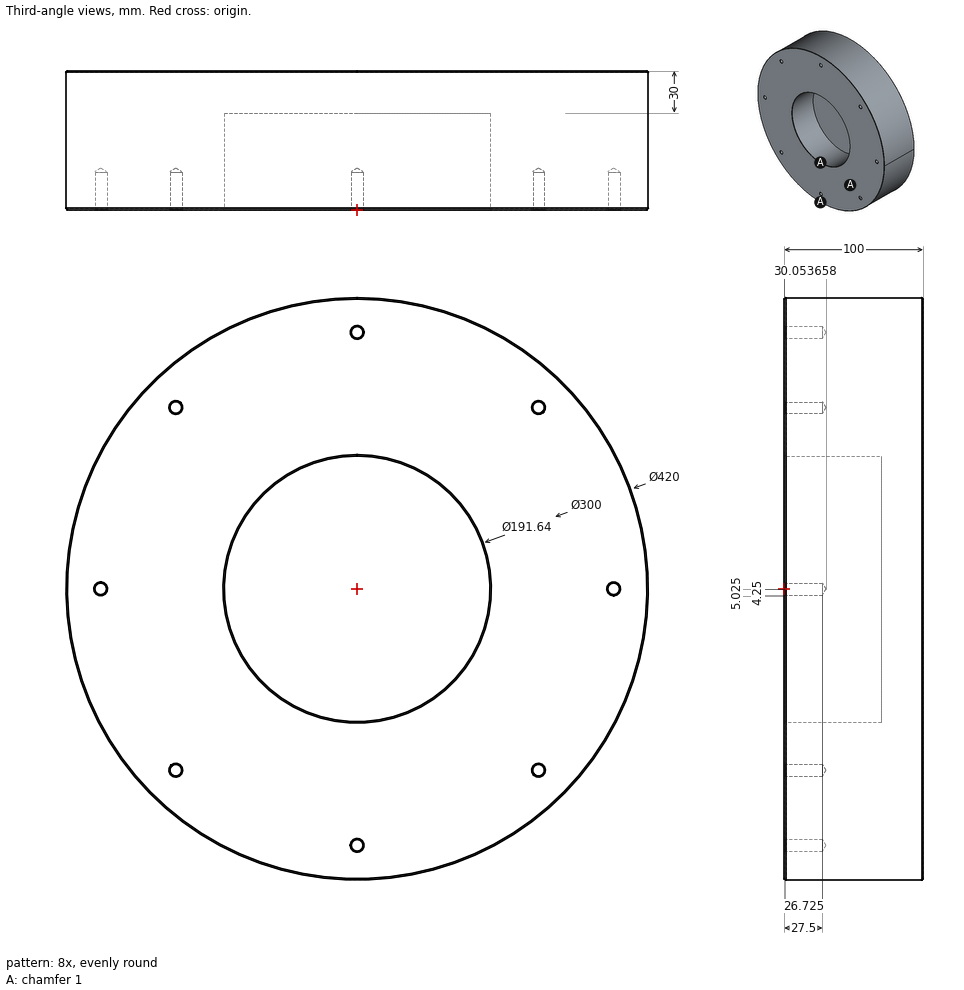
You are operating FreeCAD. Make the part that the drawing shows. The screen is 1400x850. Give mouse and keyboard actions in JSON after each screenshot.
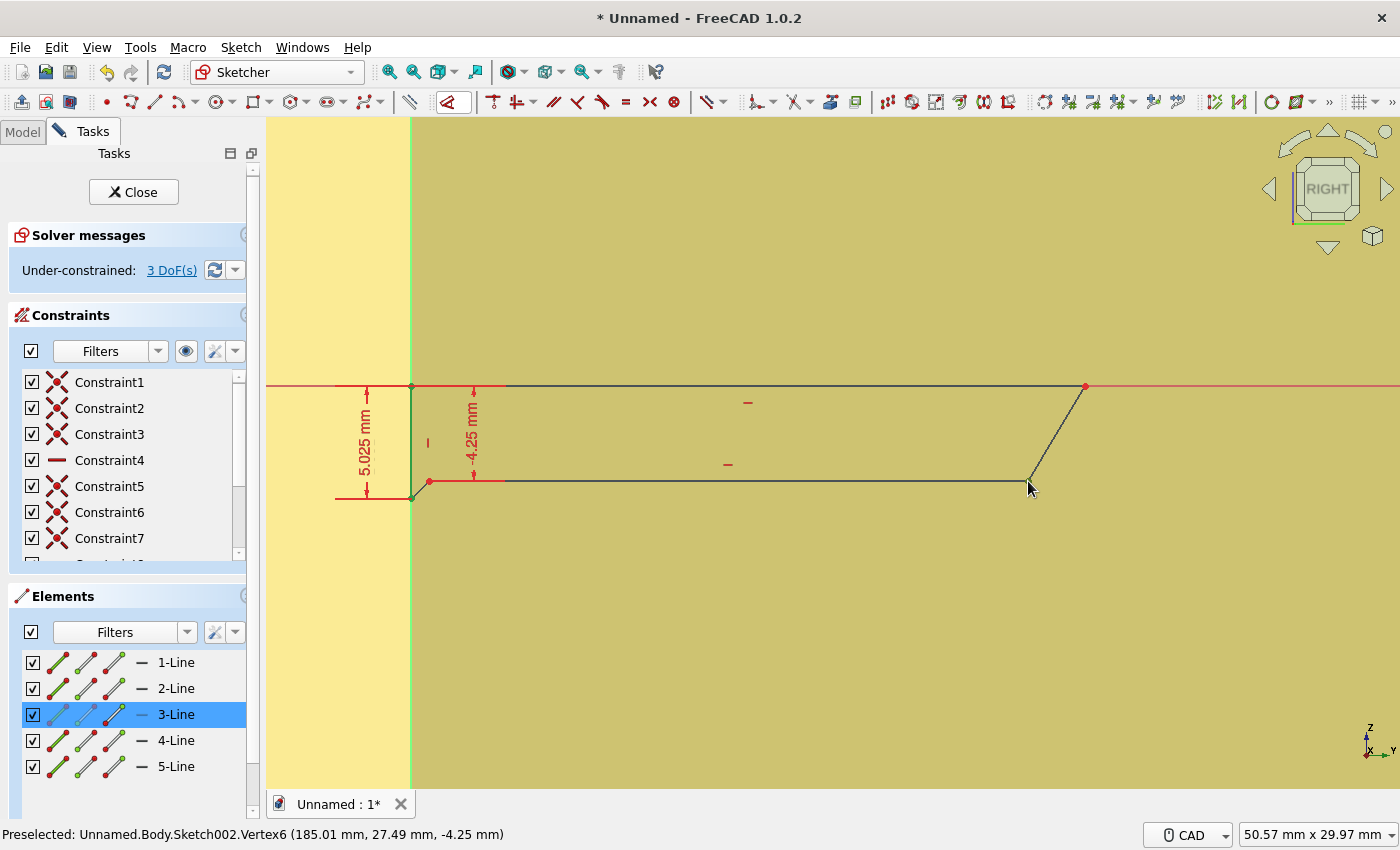
{"action": "key", "text": "l"}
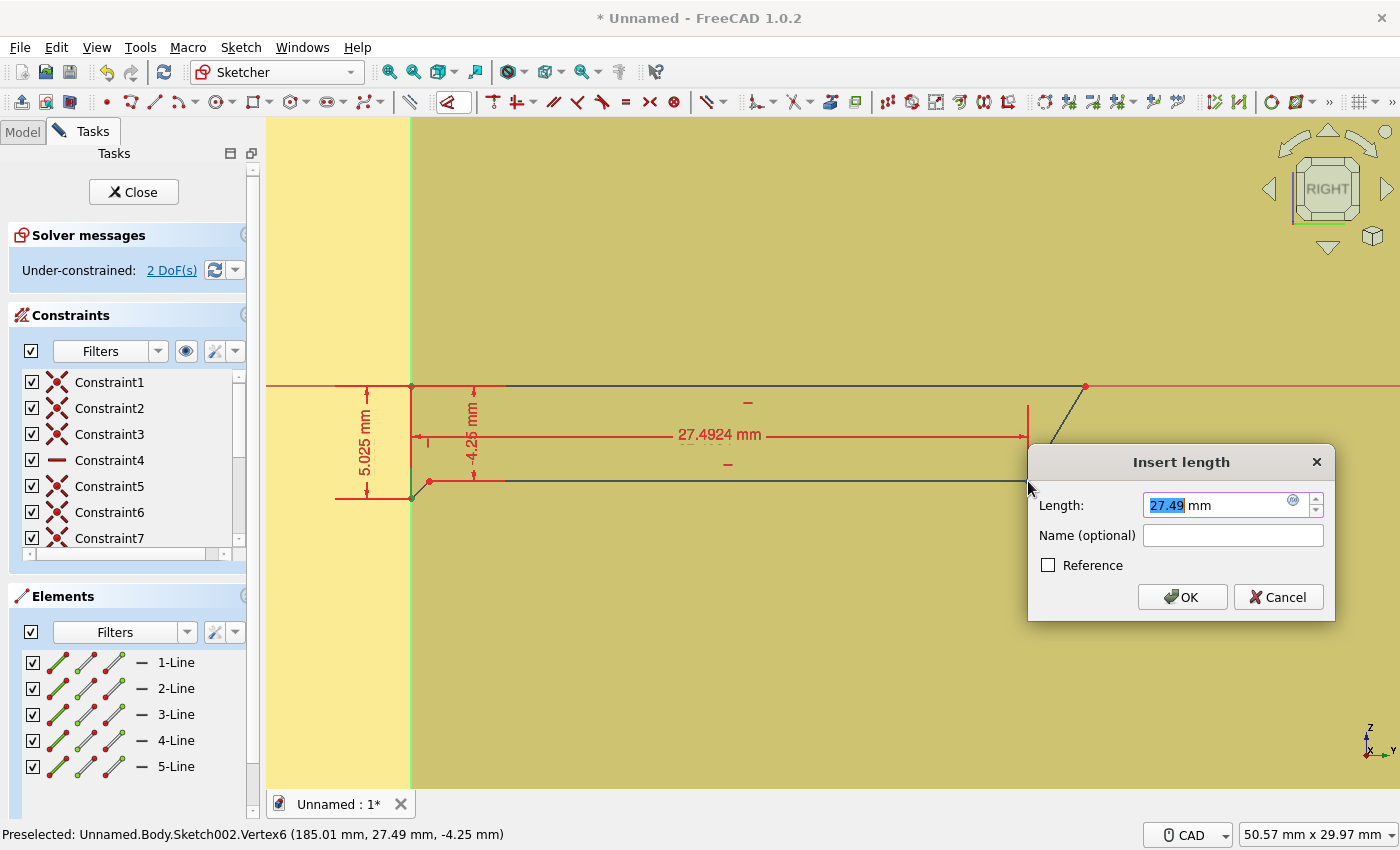
{"action": "type", "text": "27.5"}
{"action": "key", "text": "Return"}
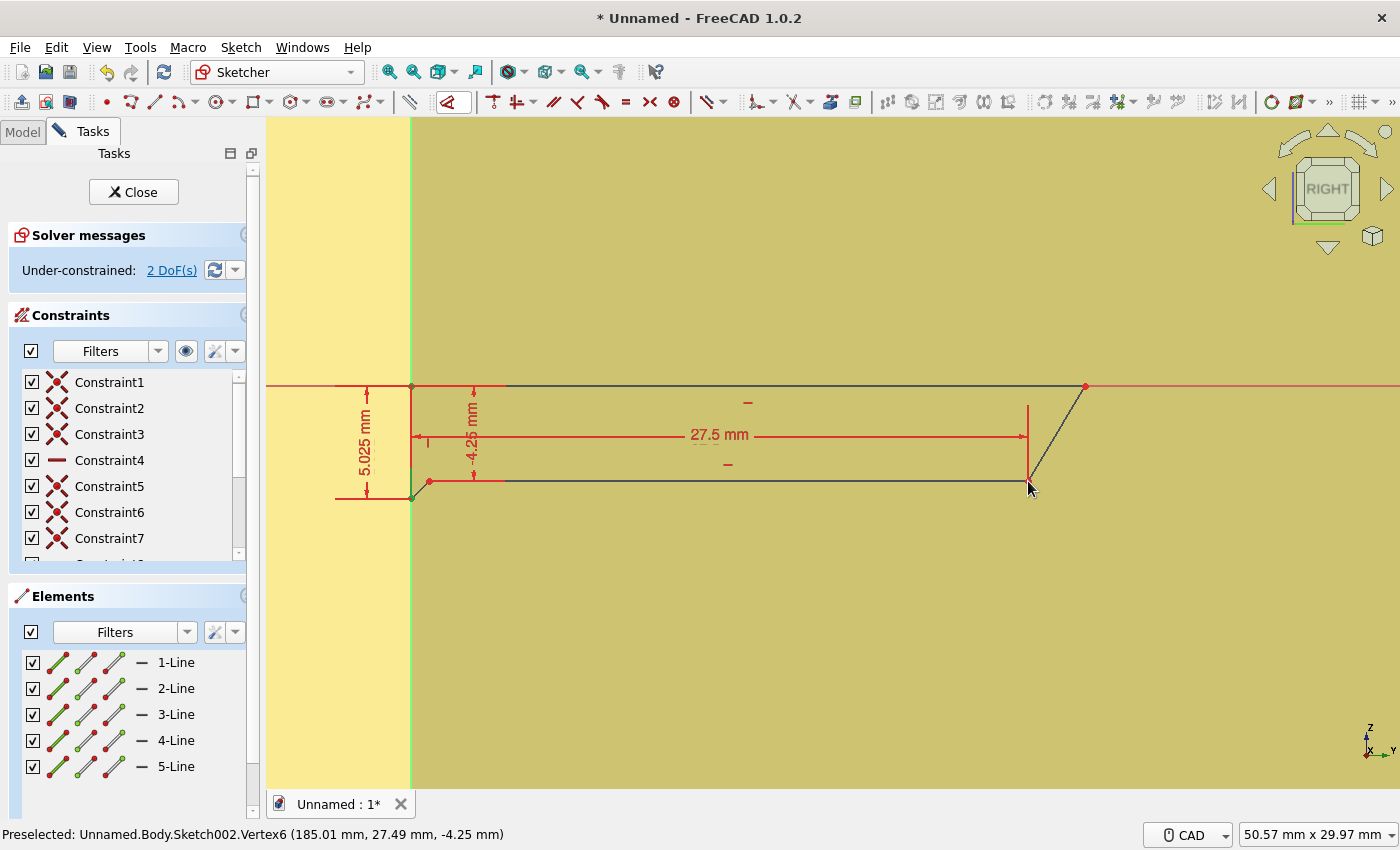
{"action": "left_click", "coordinate": [609, 481]}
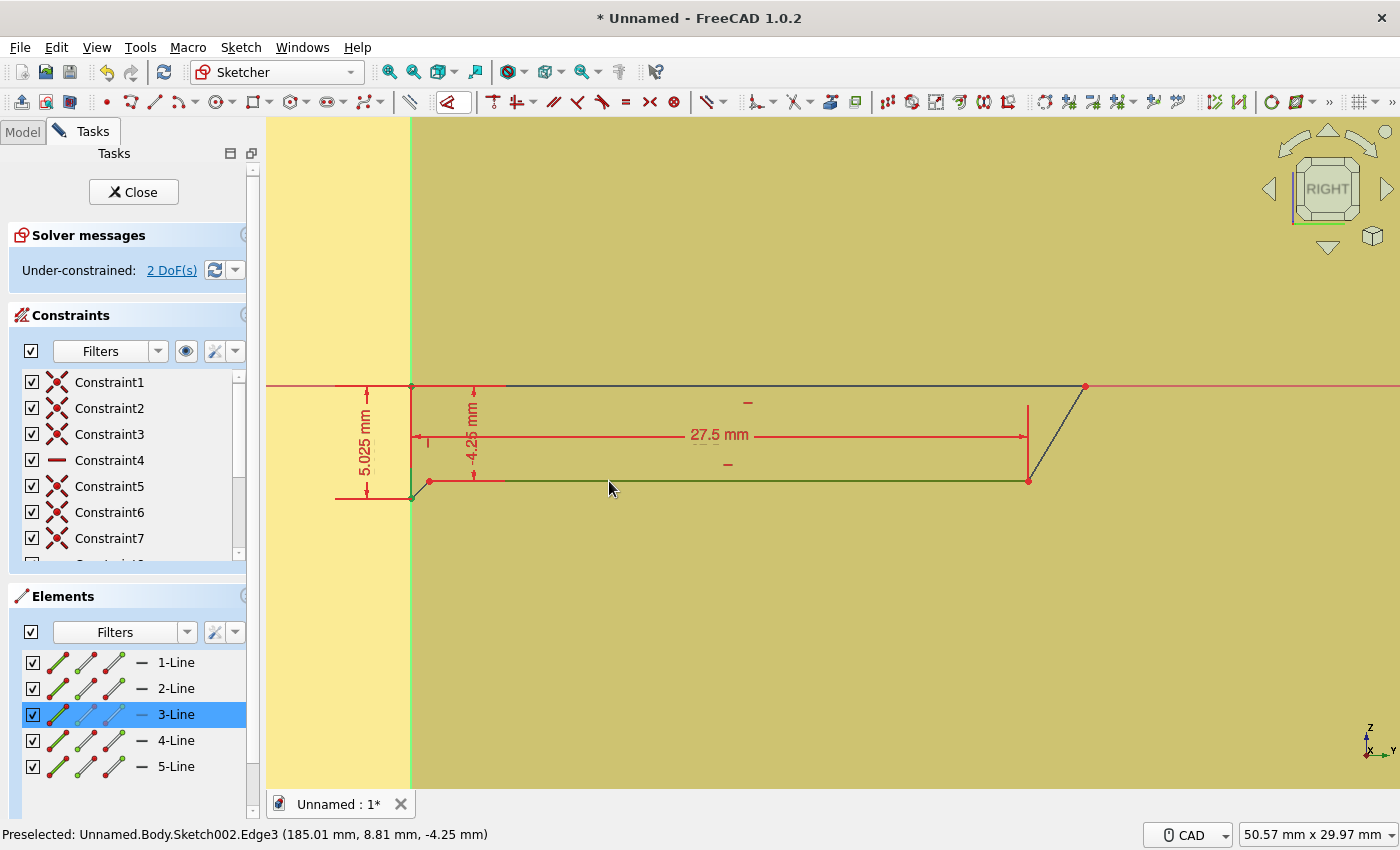
{"action": "key", "text": "l"}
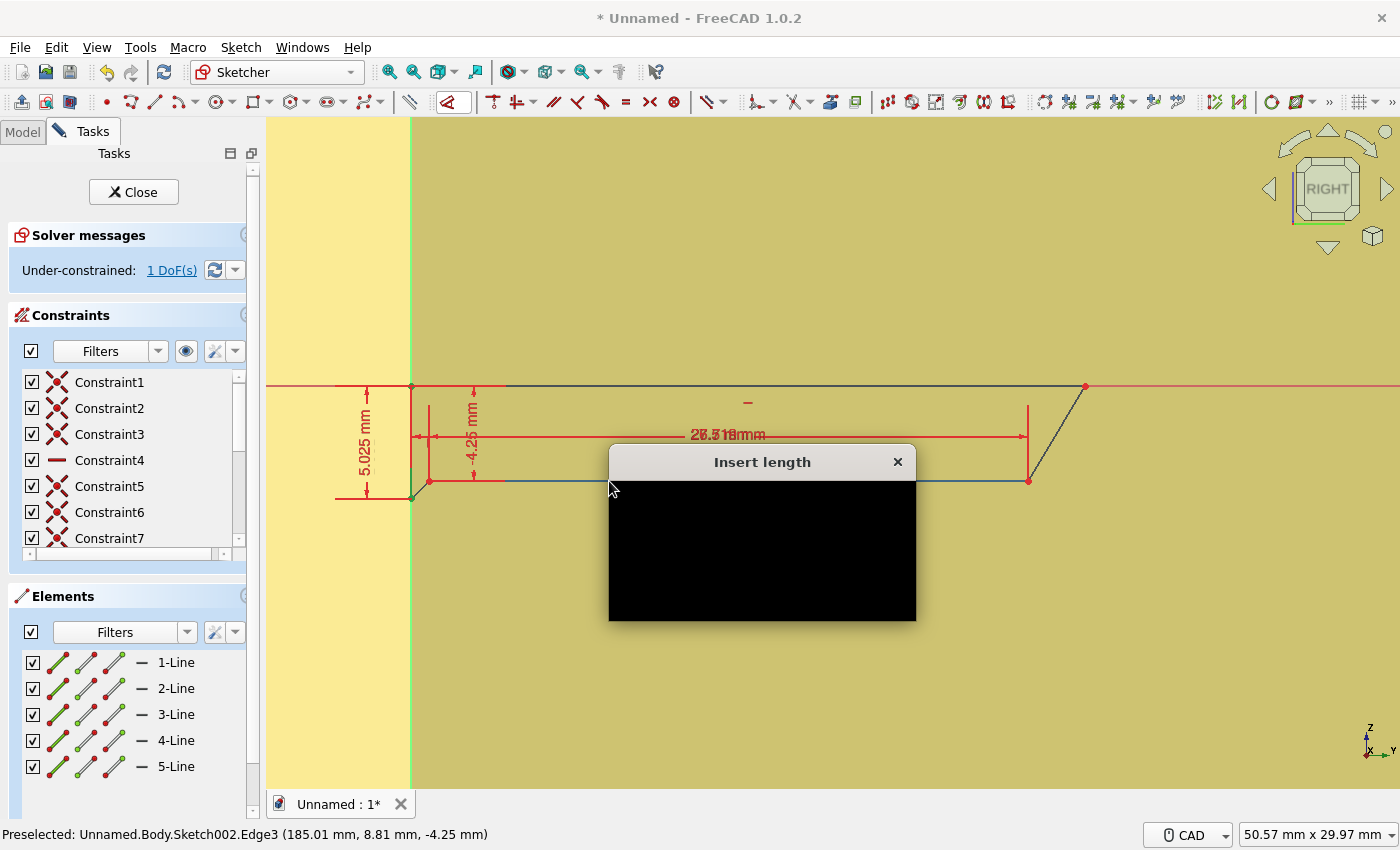
{"action": "type", "text": "26.725"}
{"action": "key", "text": "Return"}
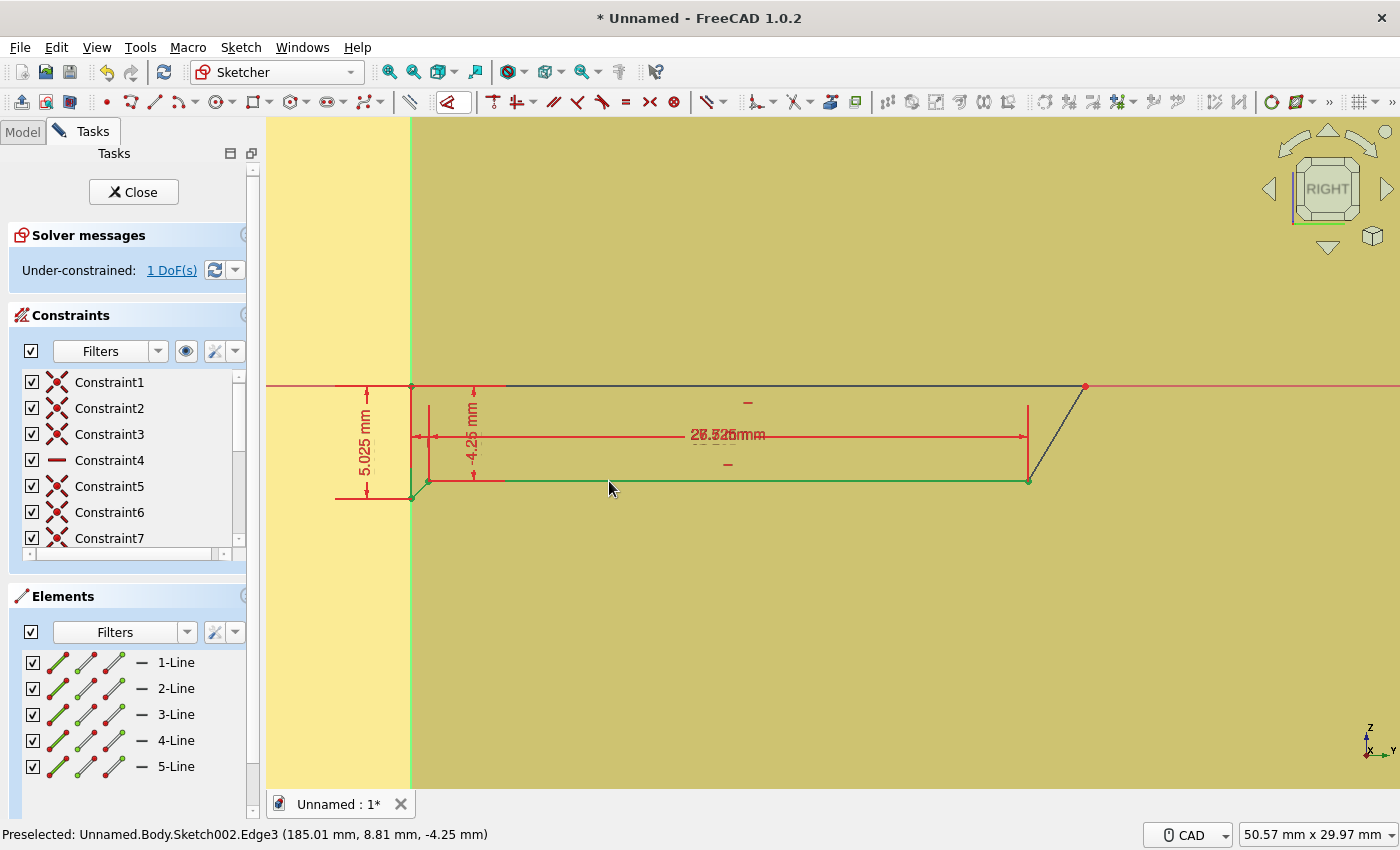
{"action": "left_click", "coordinate": [883, 386]}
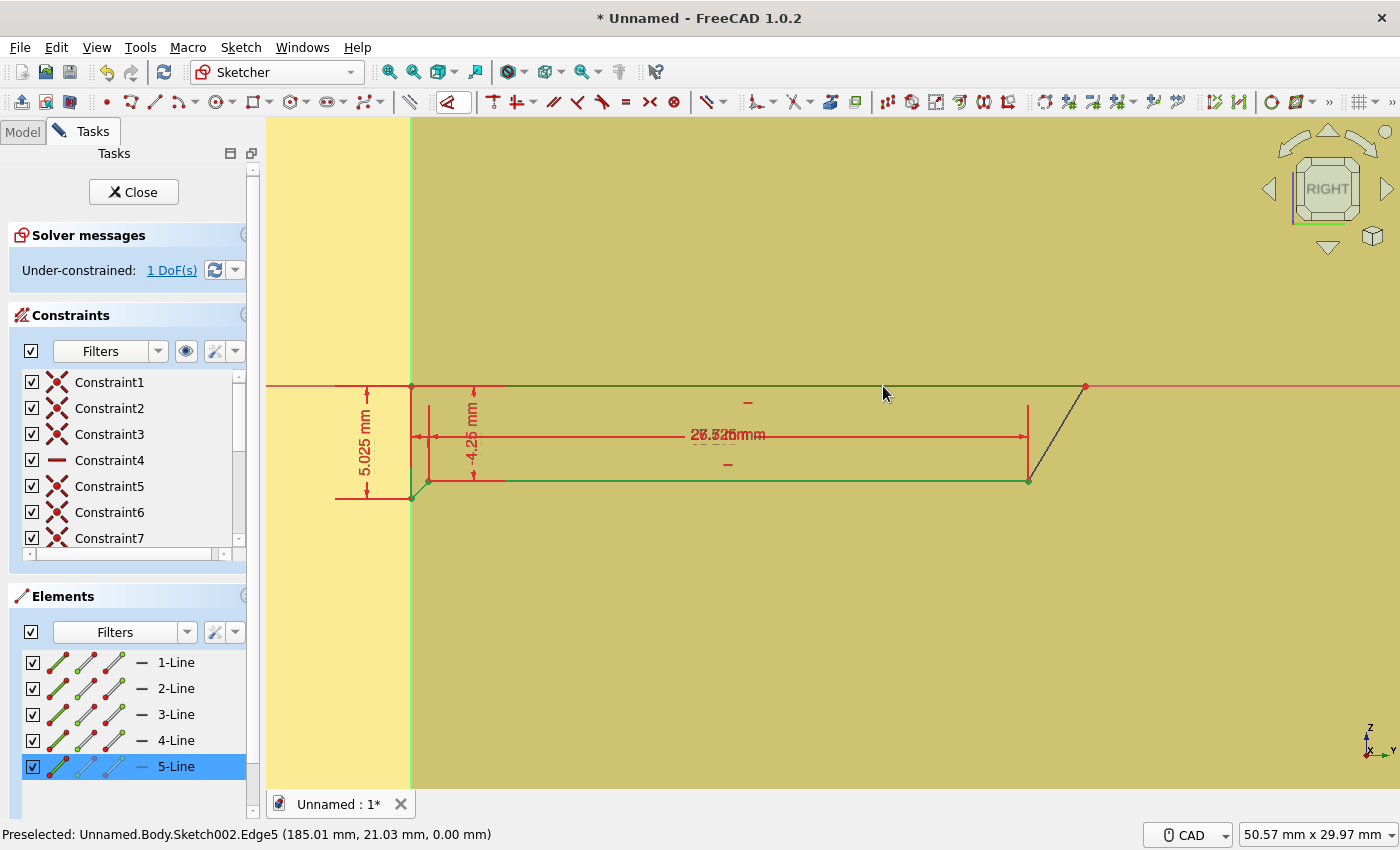
{"action": "key", "text": "l"}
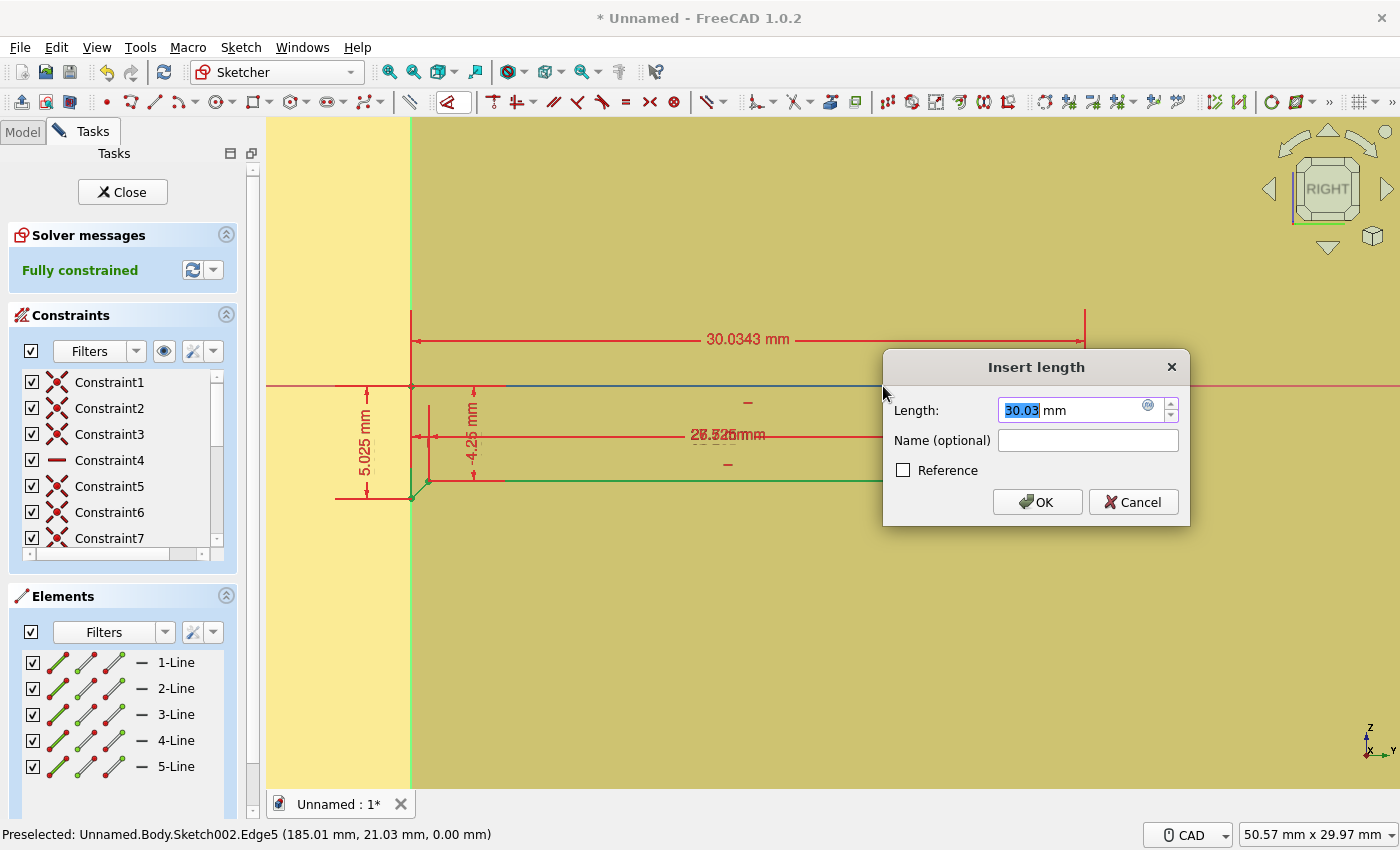
{"action": "type", "text": "30.053658"}
{"action": "key", "text": "Return"}